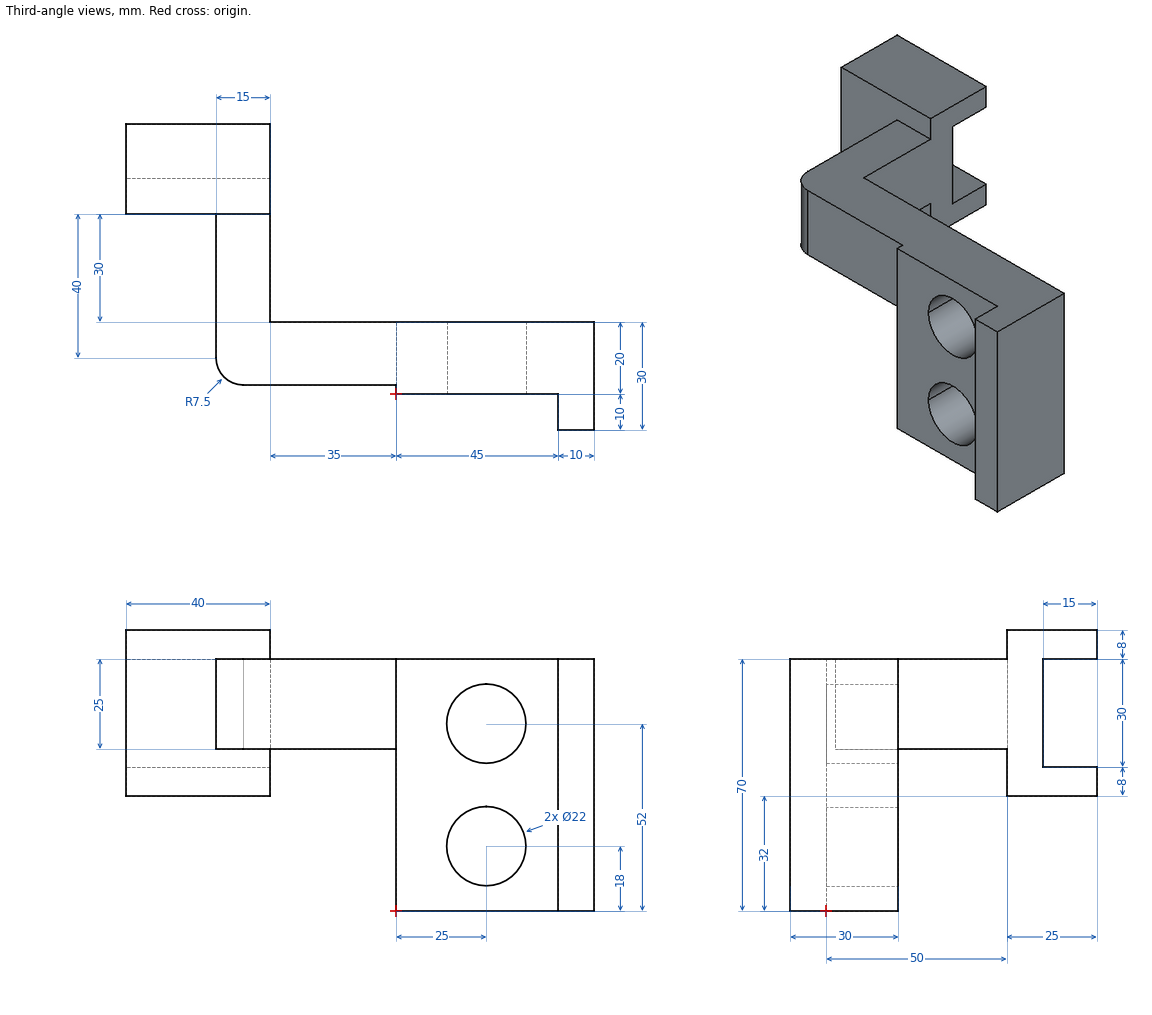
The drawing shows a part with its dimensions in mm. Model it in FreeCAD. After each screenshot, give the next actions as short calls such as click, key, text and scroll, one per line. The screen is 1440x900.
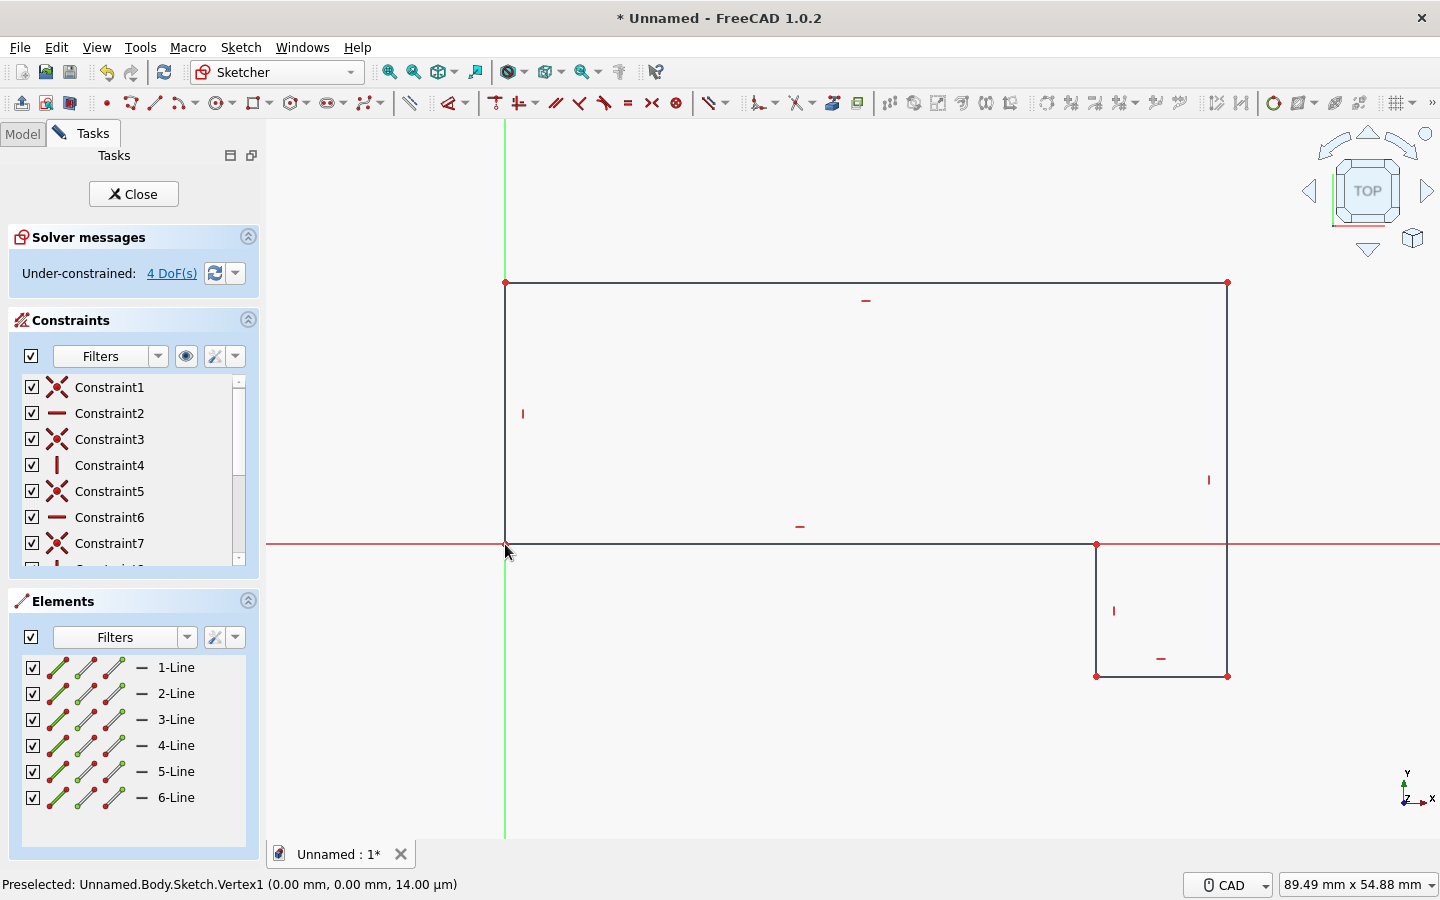
key(d)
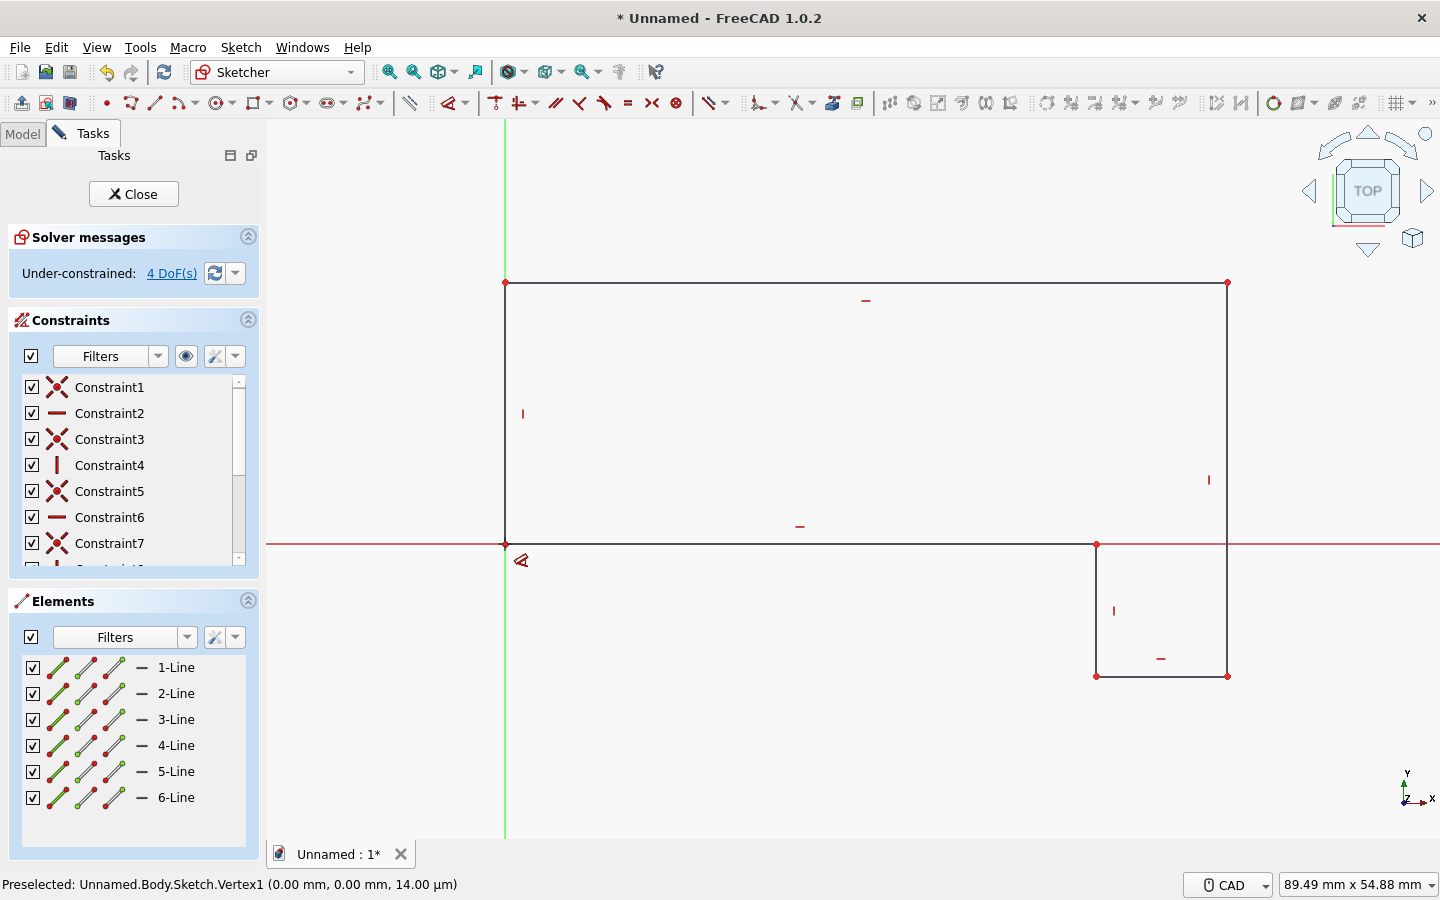
click(683, 544)
click(801, 578)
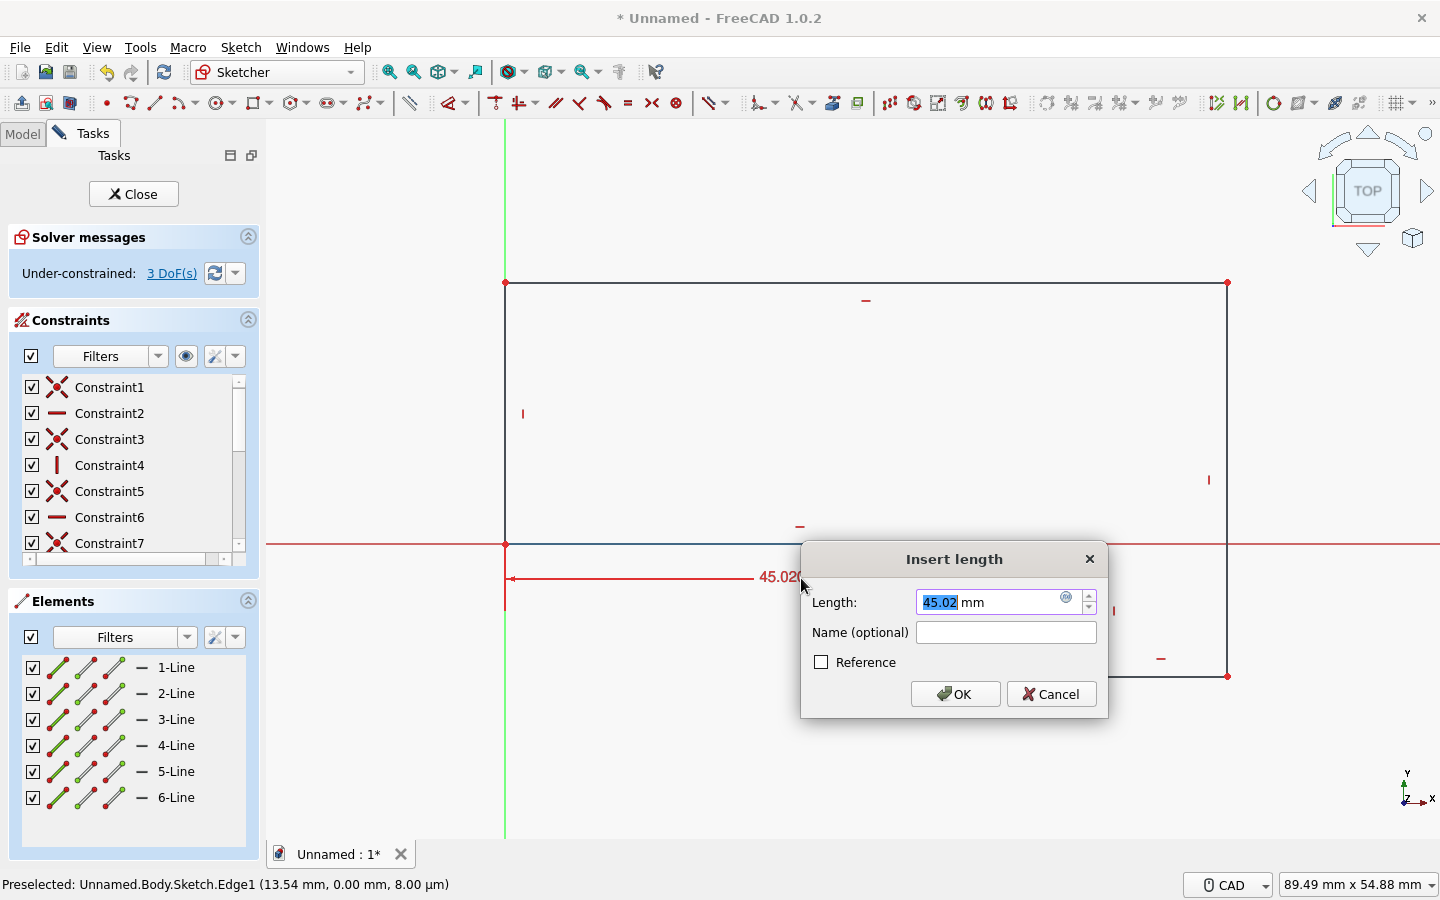
text(45)
key(Return)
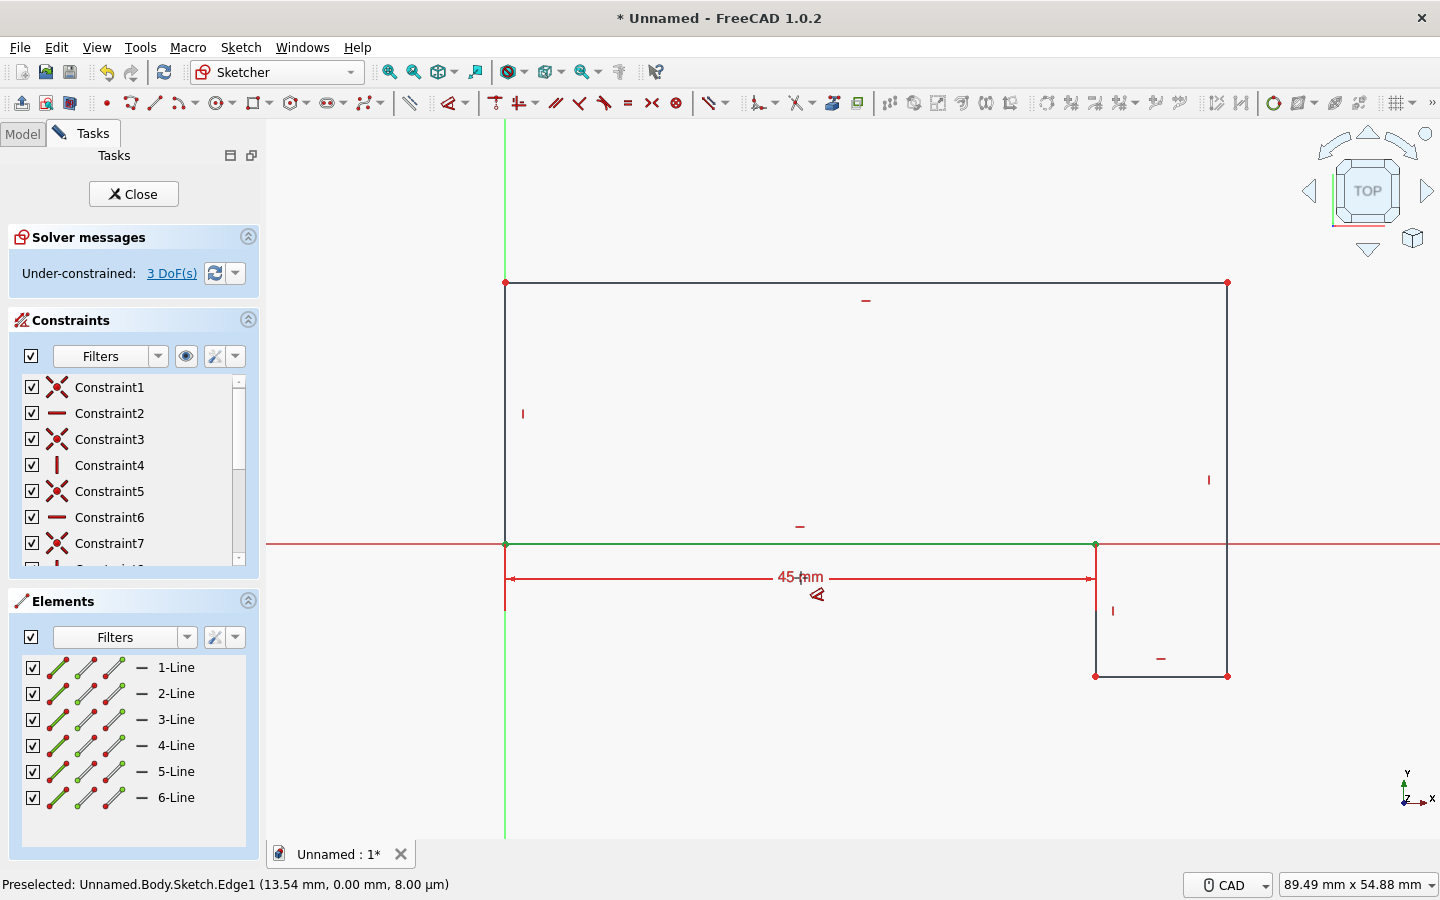
click(1096, 584)
click(1130, 611)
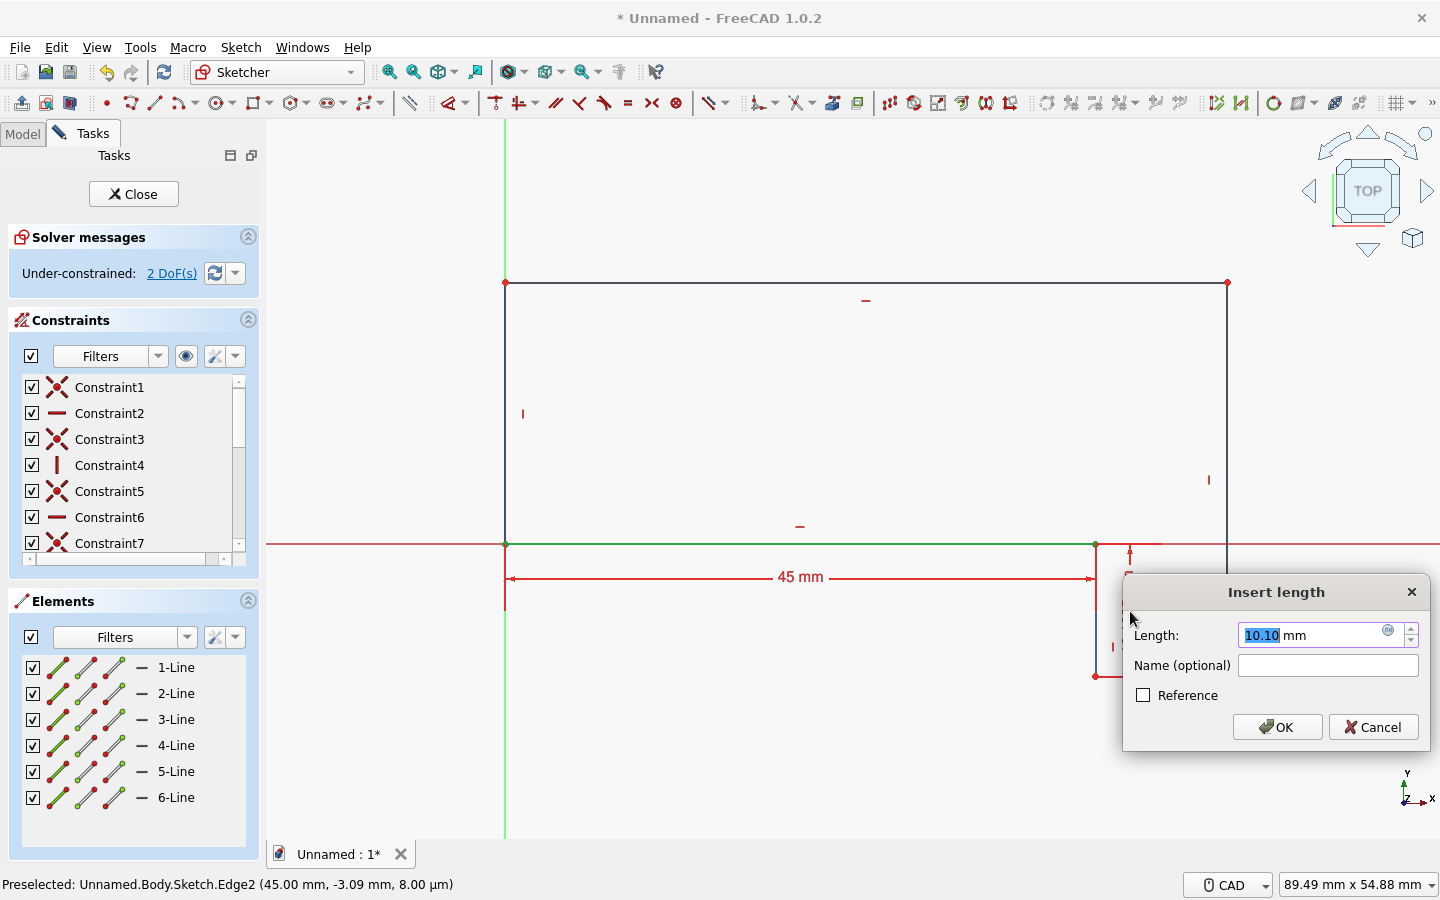
text(10)
key(Return)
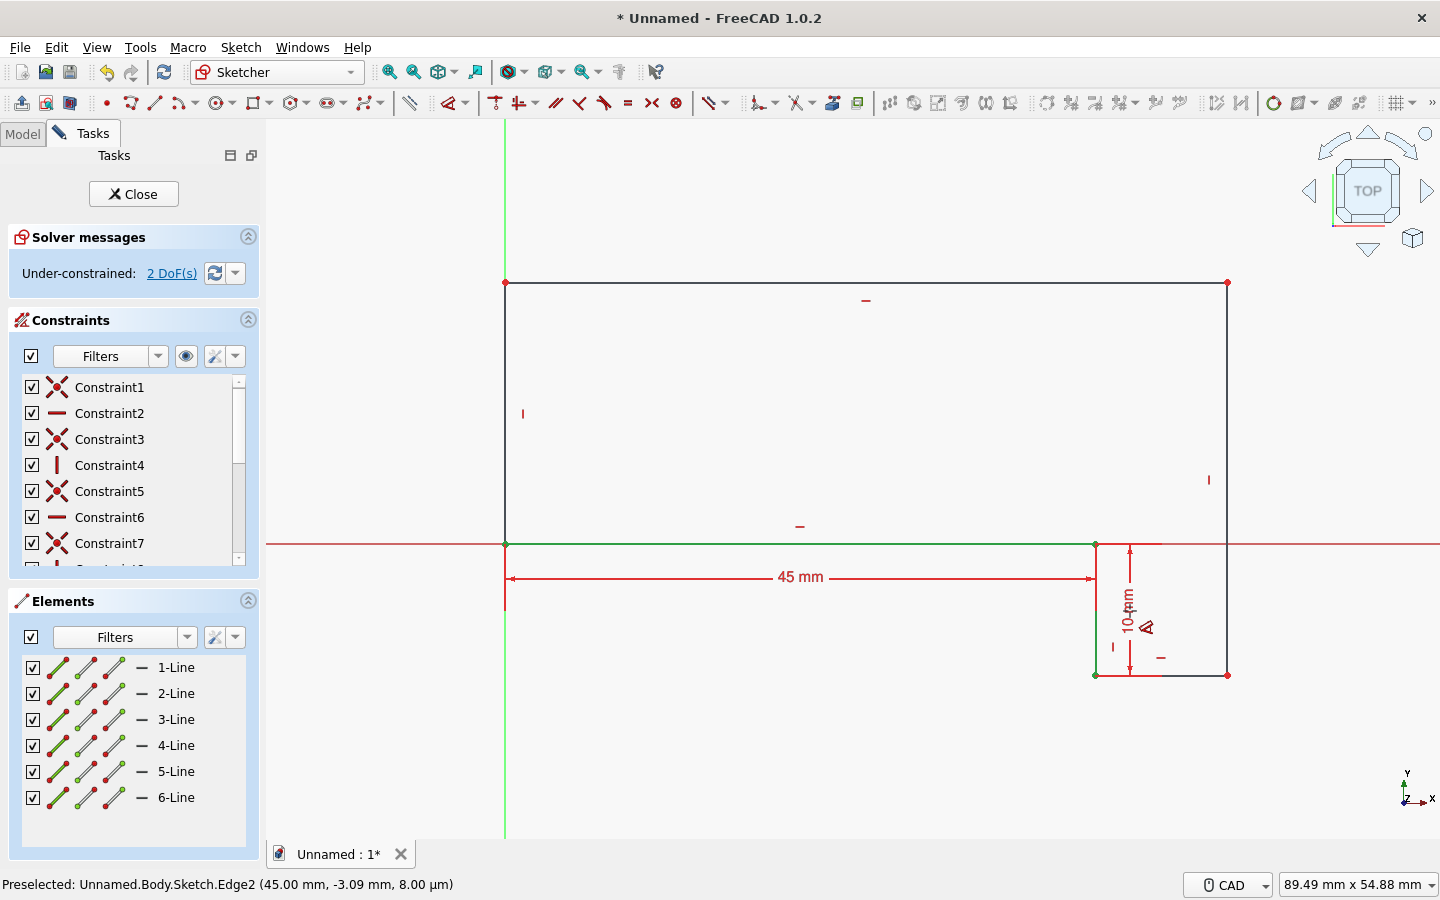
click(1135, 676)
click(1161, 710)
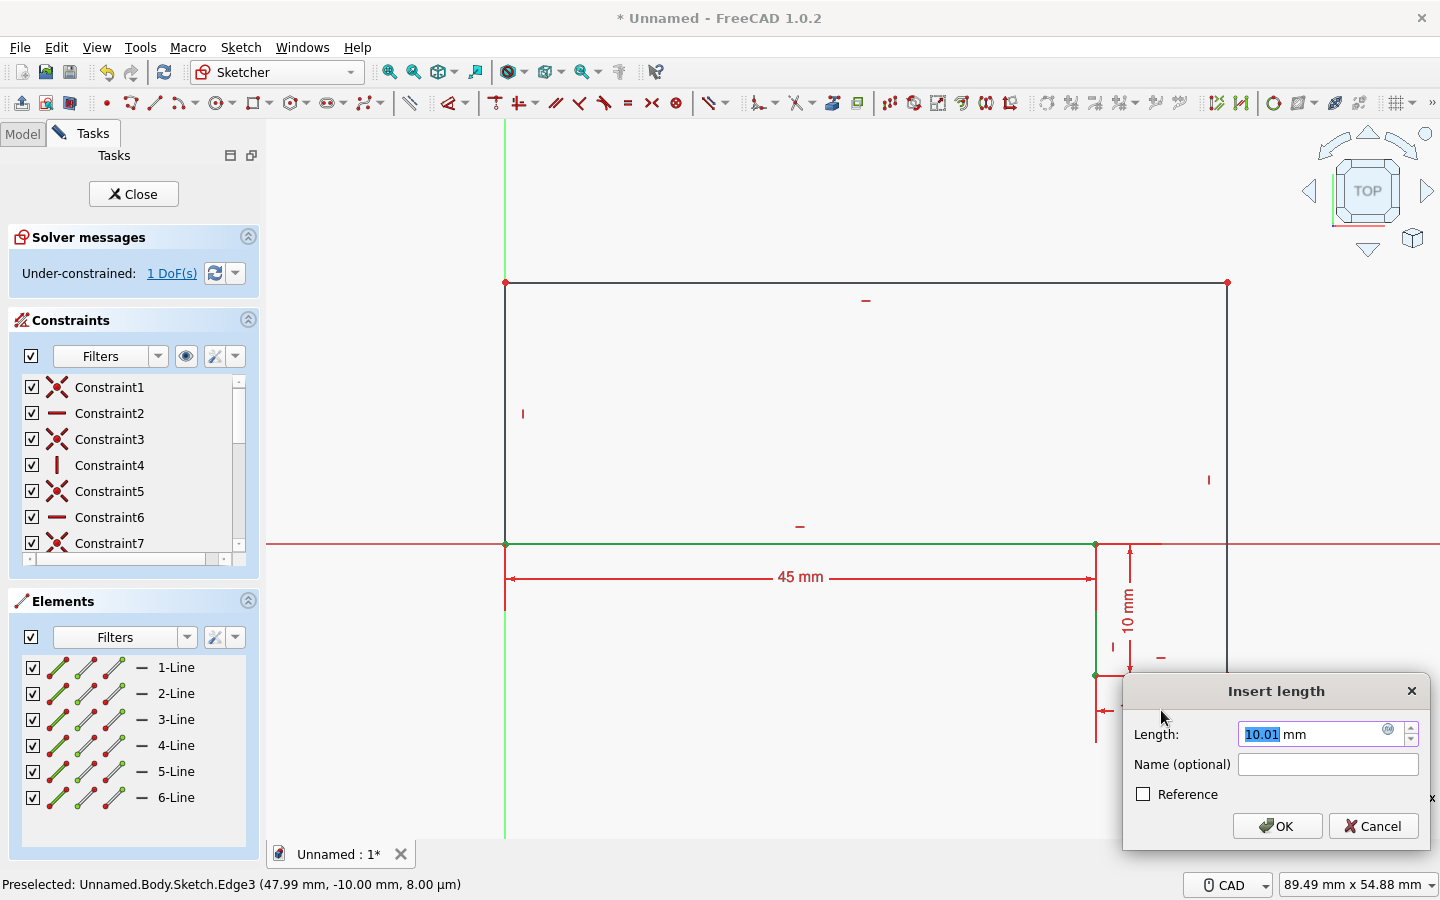
text(10)
key(Return)